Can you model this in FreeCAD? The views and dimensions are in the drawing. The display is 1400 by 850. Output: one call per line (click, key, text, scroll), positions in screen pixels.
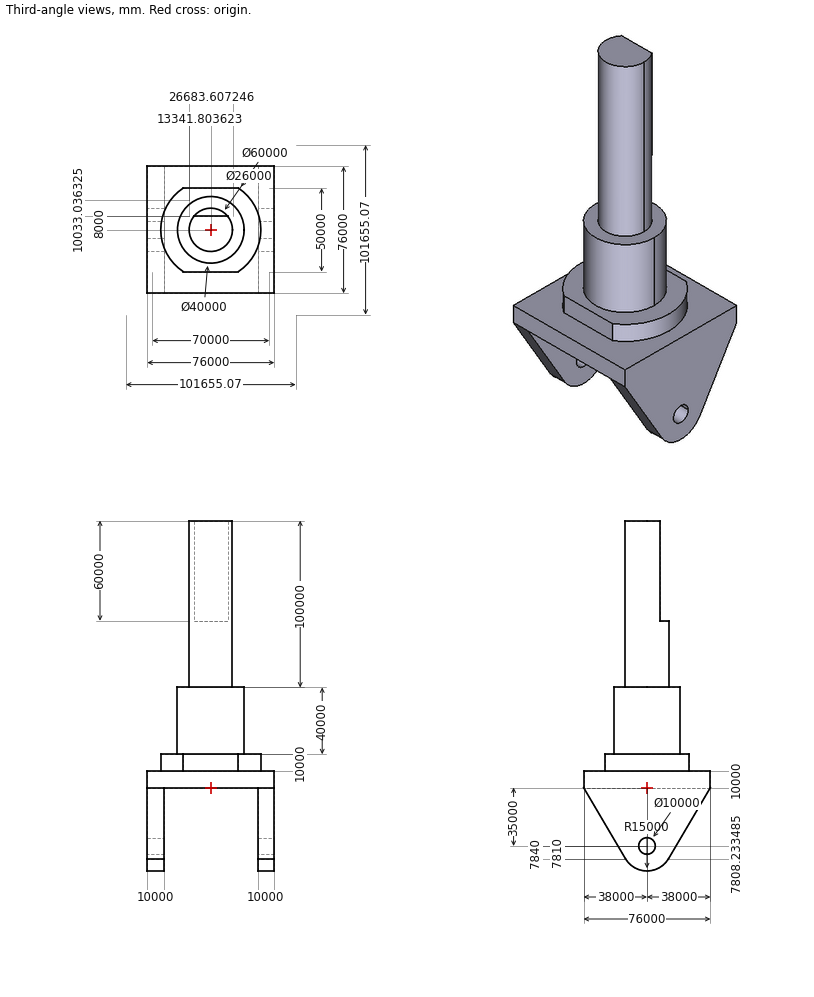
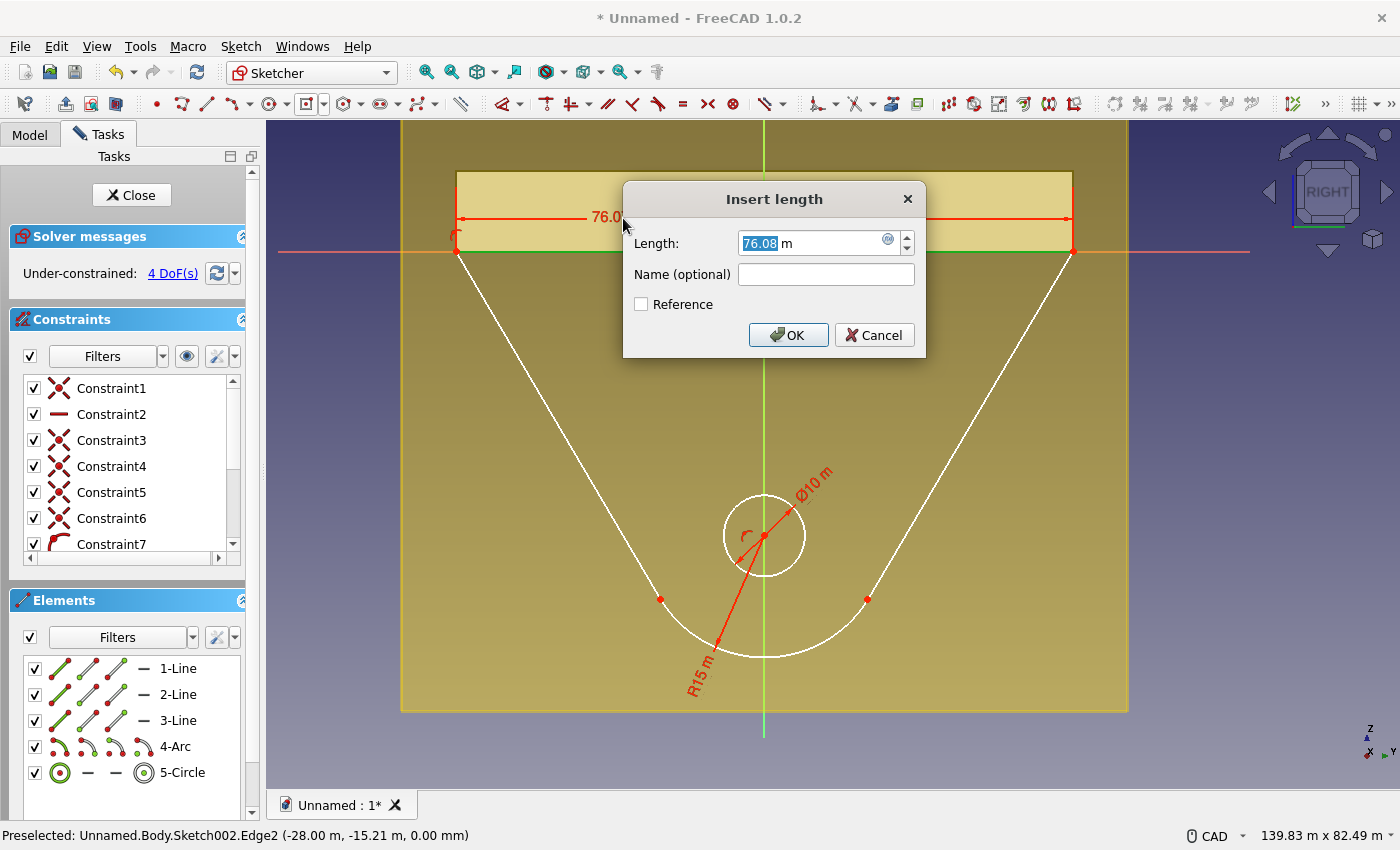
key(ctrl+a)
text(76000 mm)
key(Return)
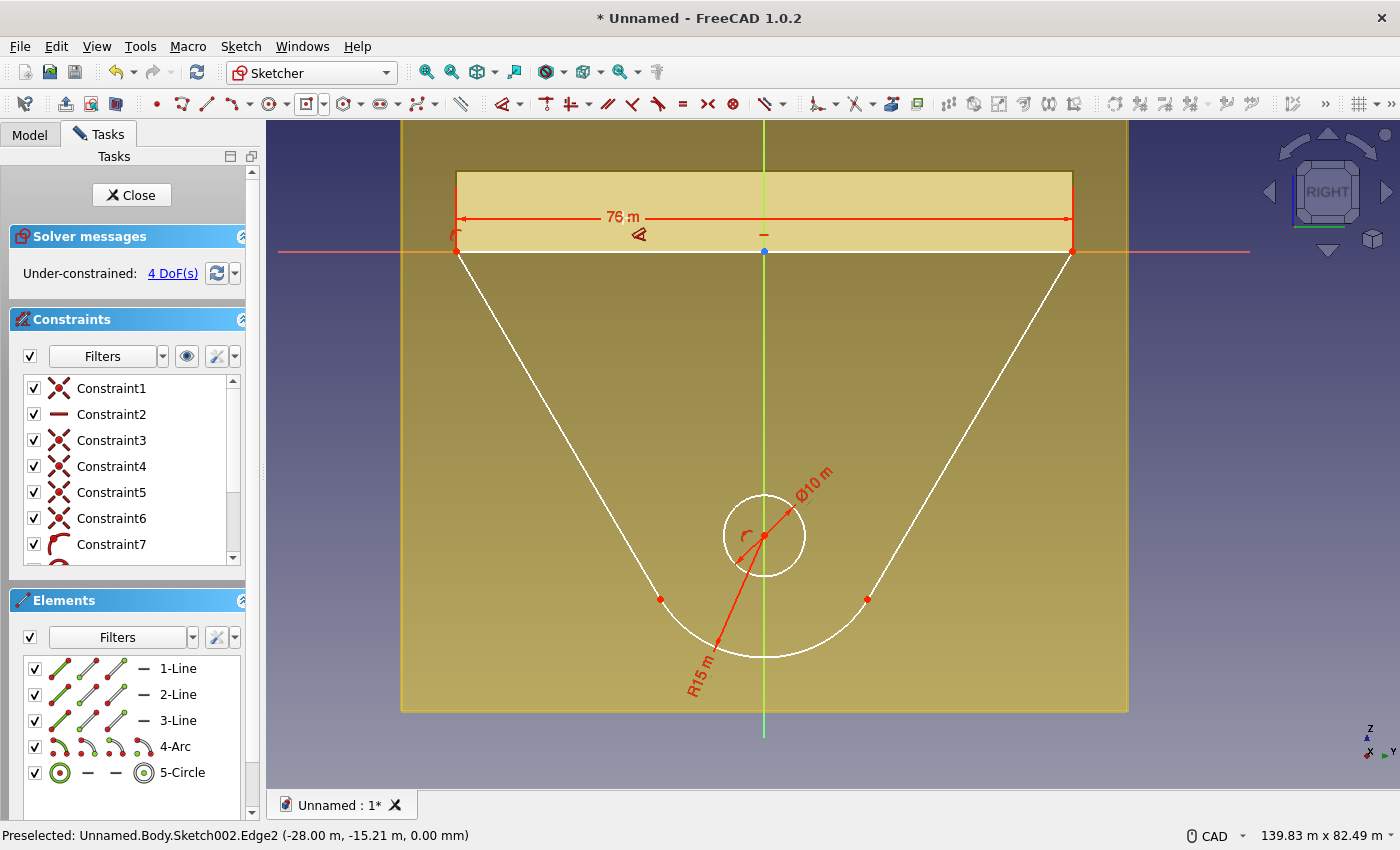
click(764, 536)
click(798, 394)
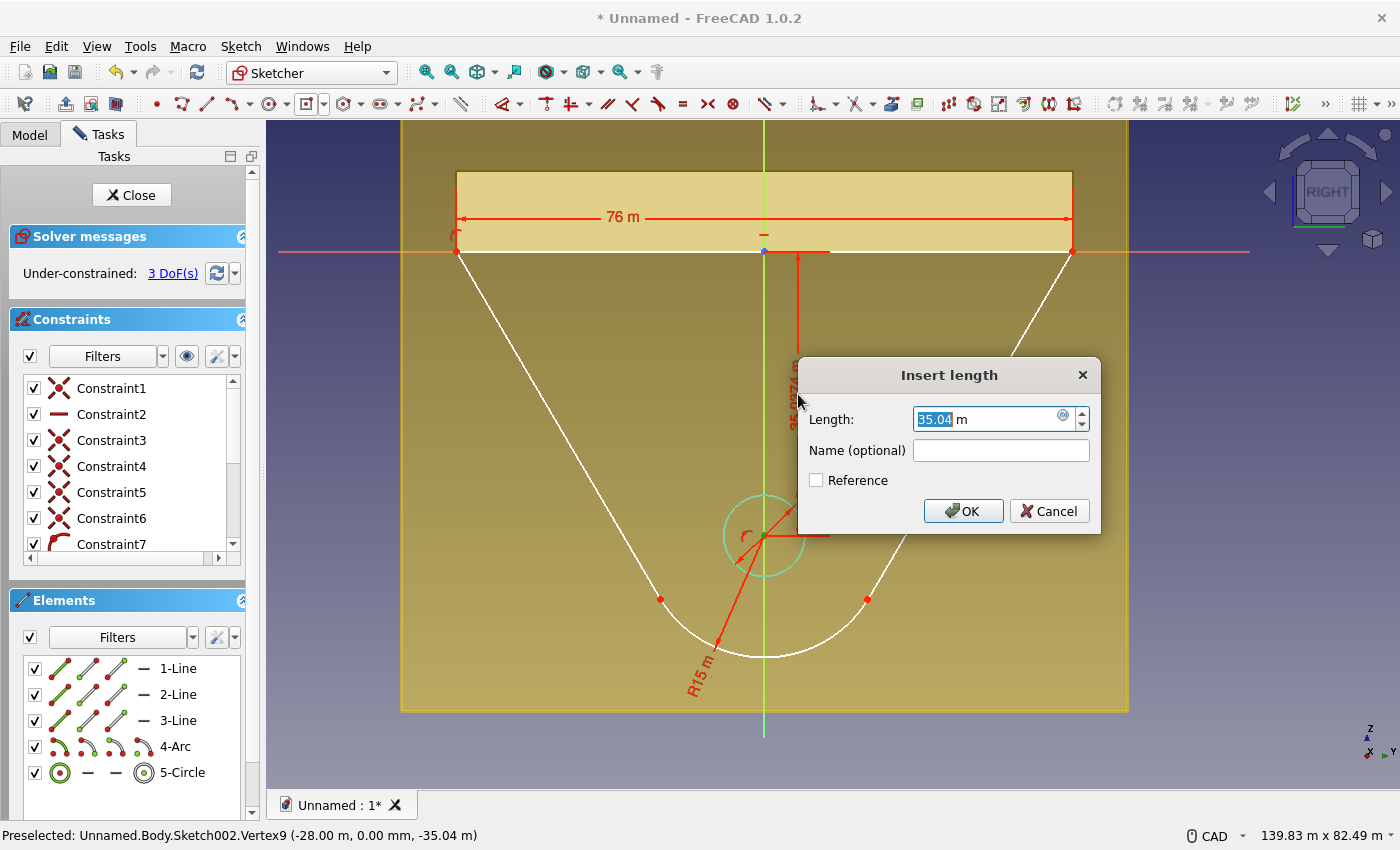
key(ctrl+a)
text(35000 mm)
key(Return)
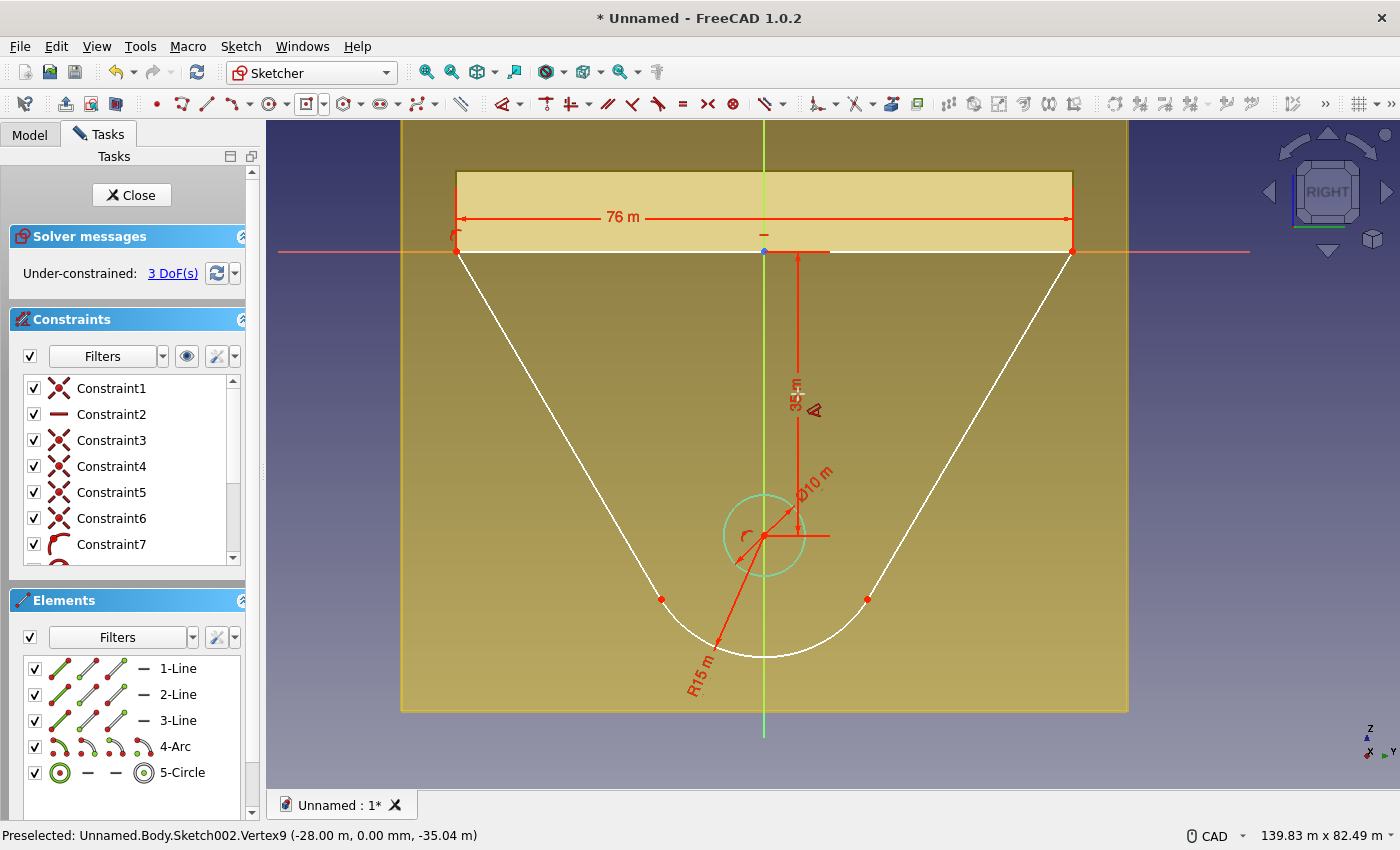
click(661, 600)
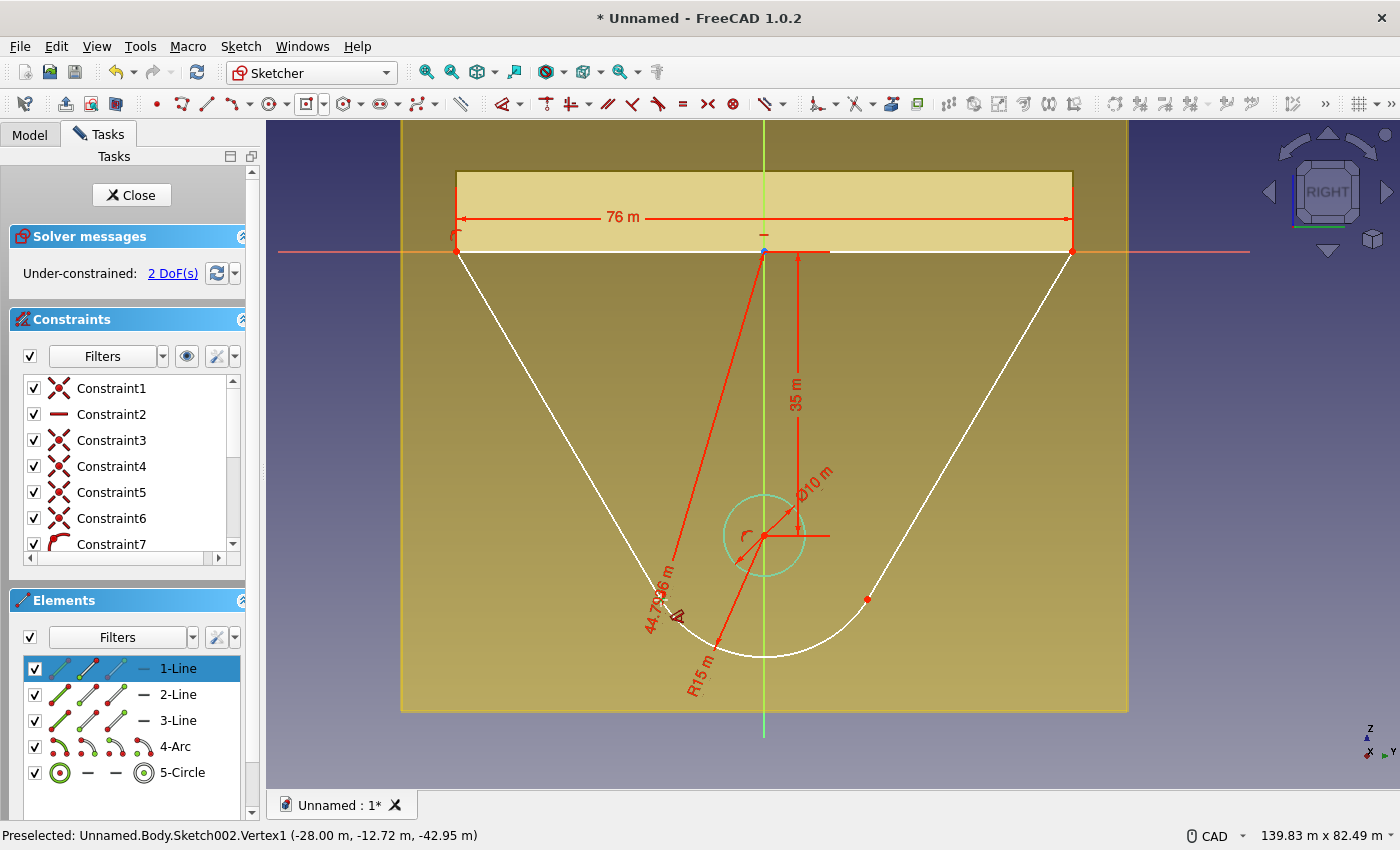
click(764, 536)
click(627, 583)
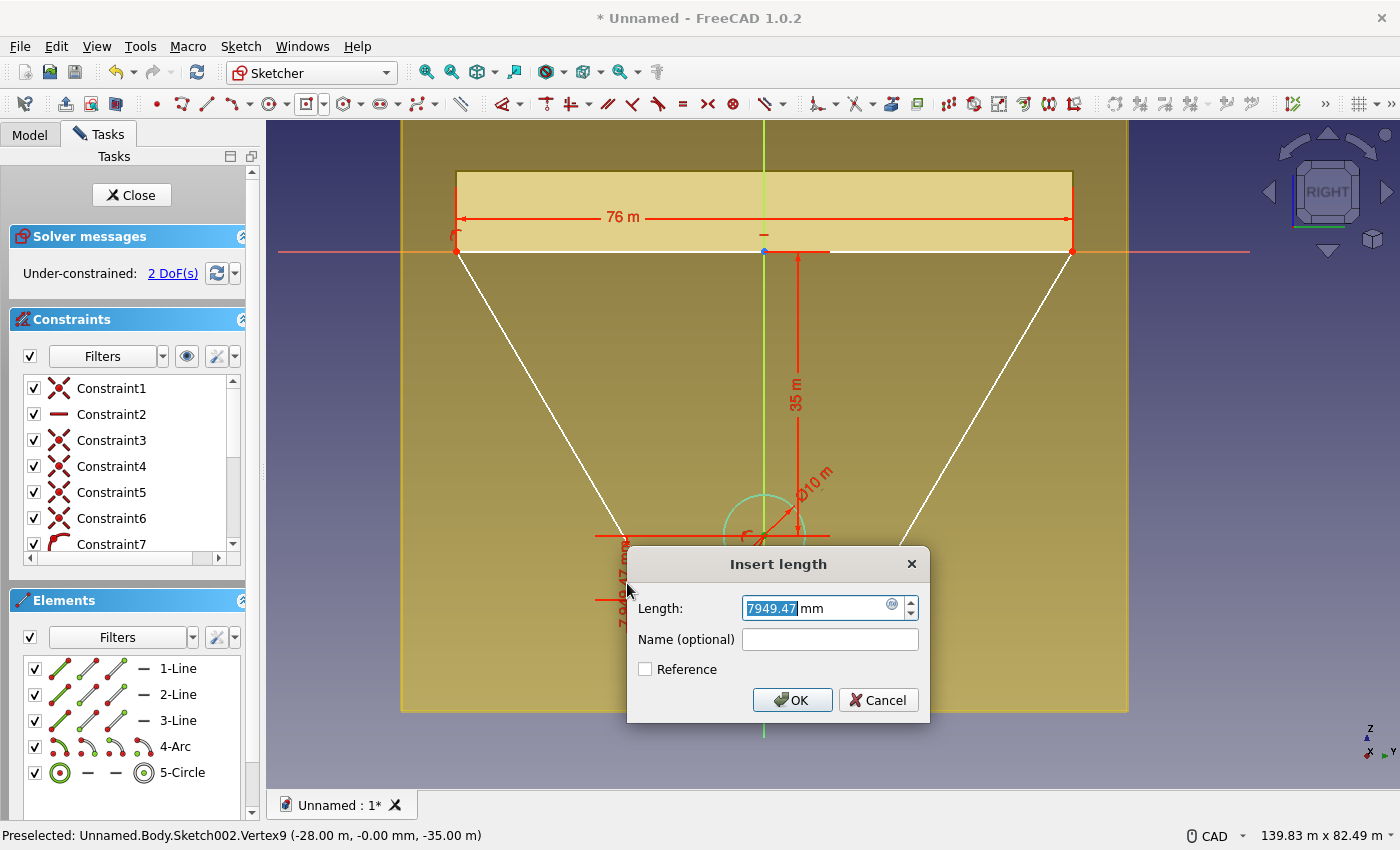
text(7840)
key(Return)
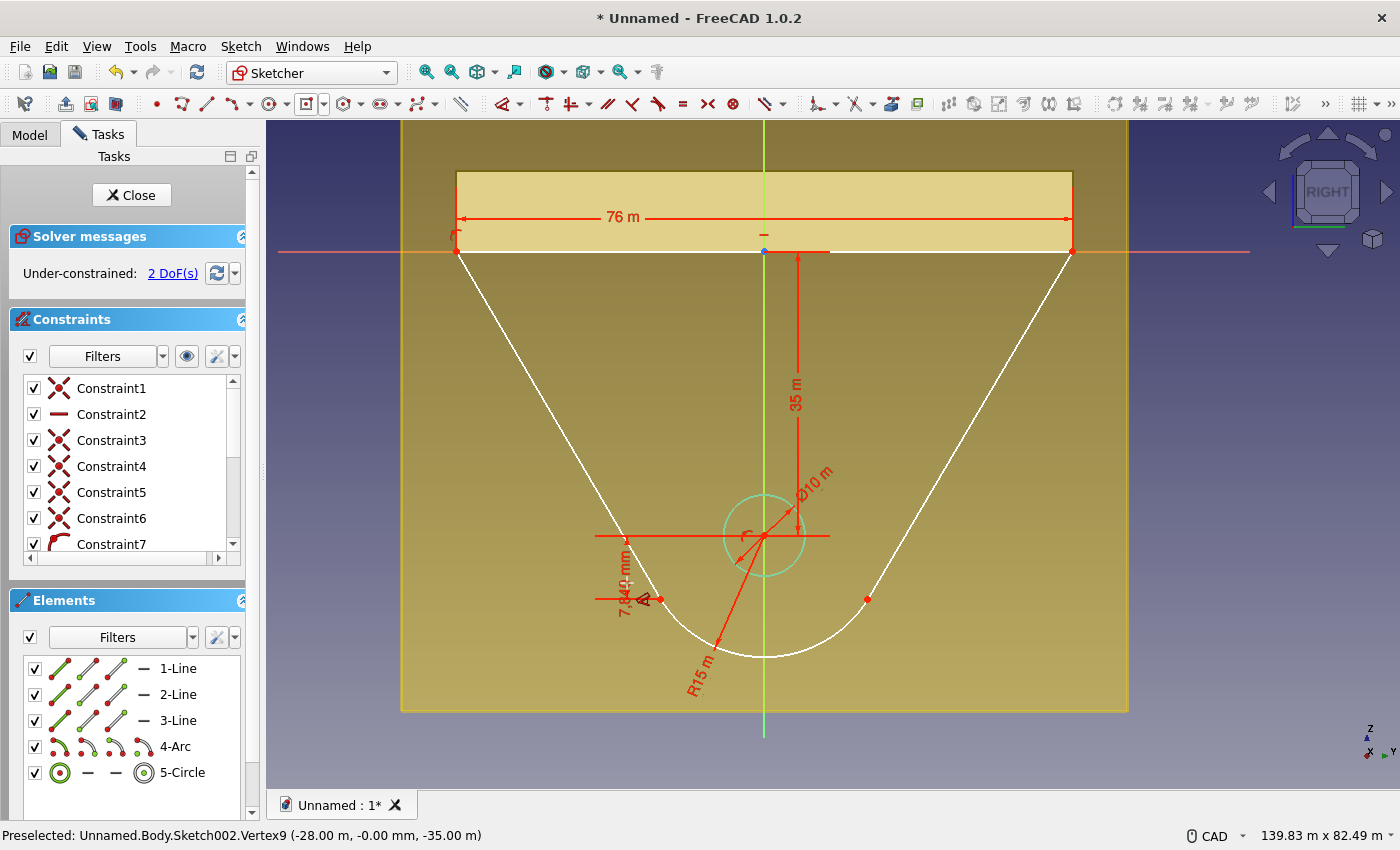
click(867, 600)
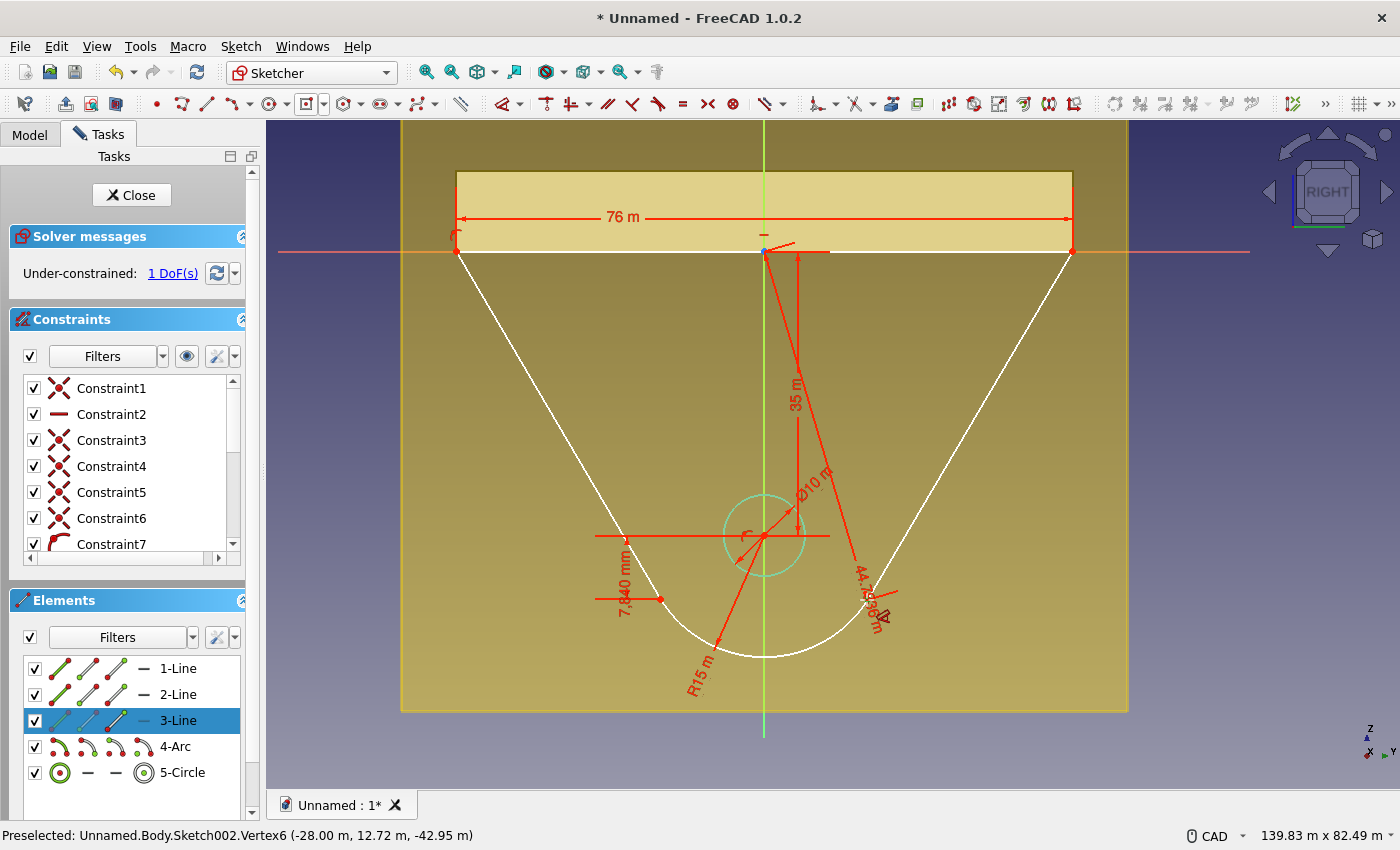
click(764, 536)
click(901, 583)